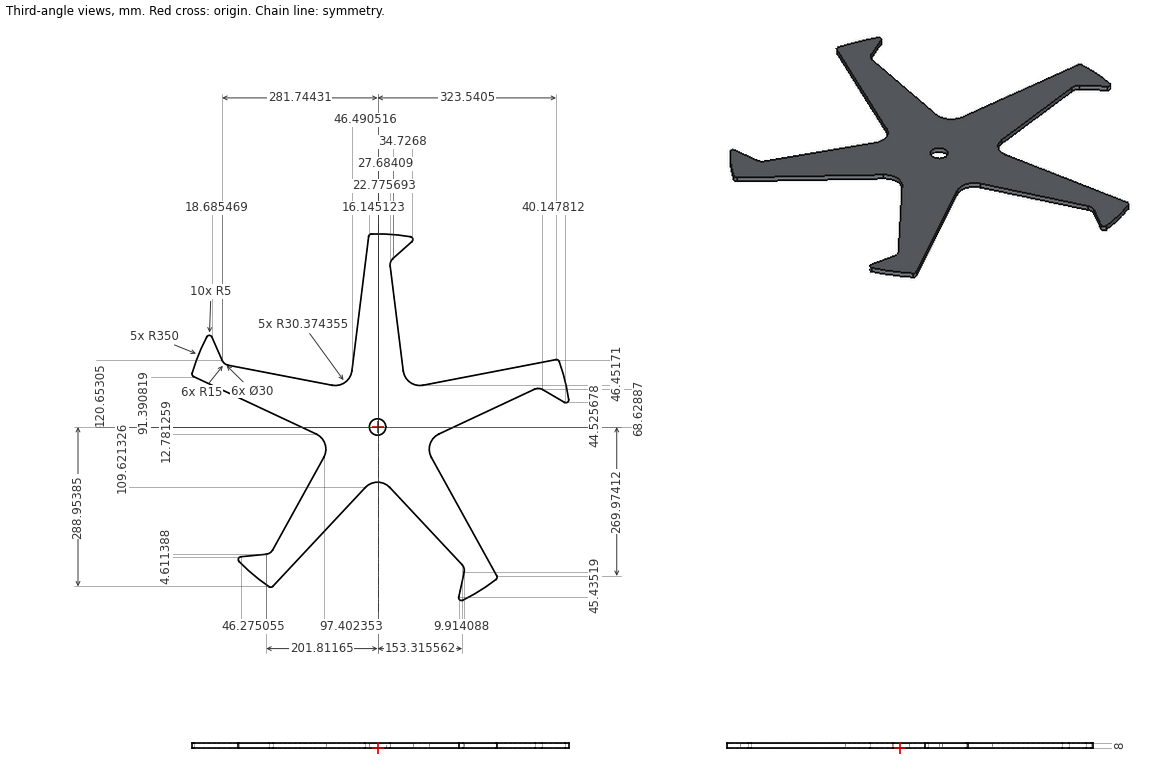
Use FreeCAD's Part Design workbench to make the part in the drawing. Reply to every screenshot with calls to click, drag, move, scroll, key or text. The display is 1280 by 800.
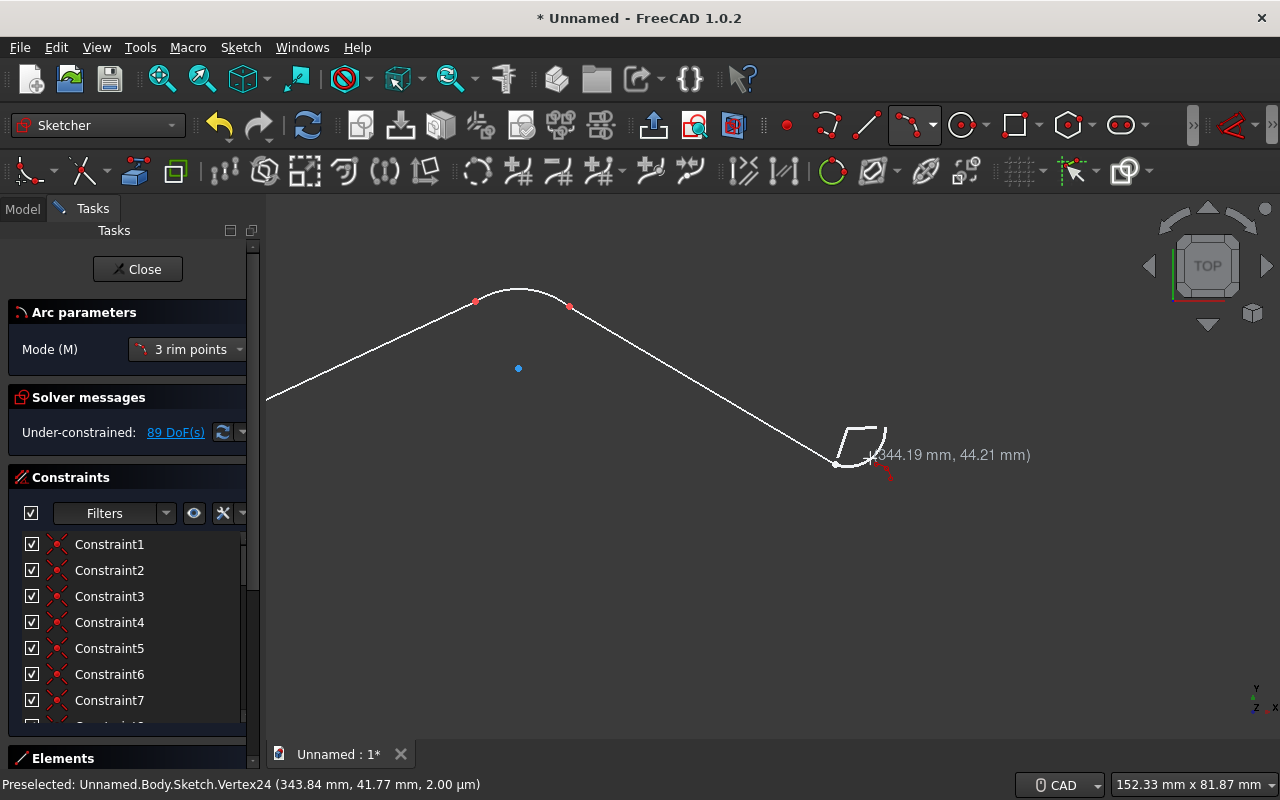
click(869, 457)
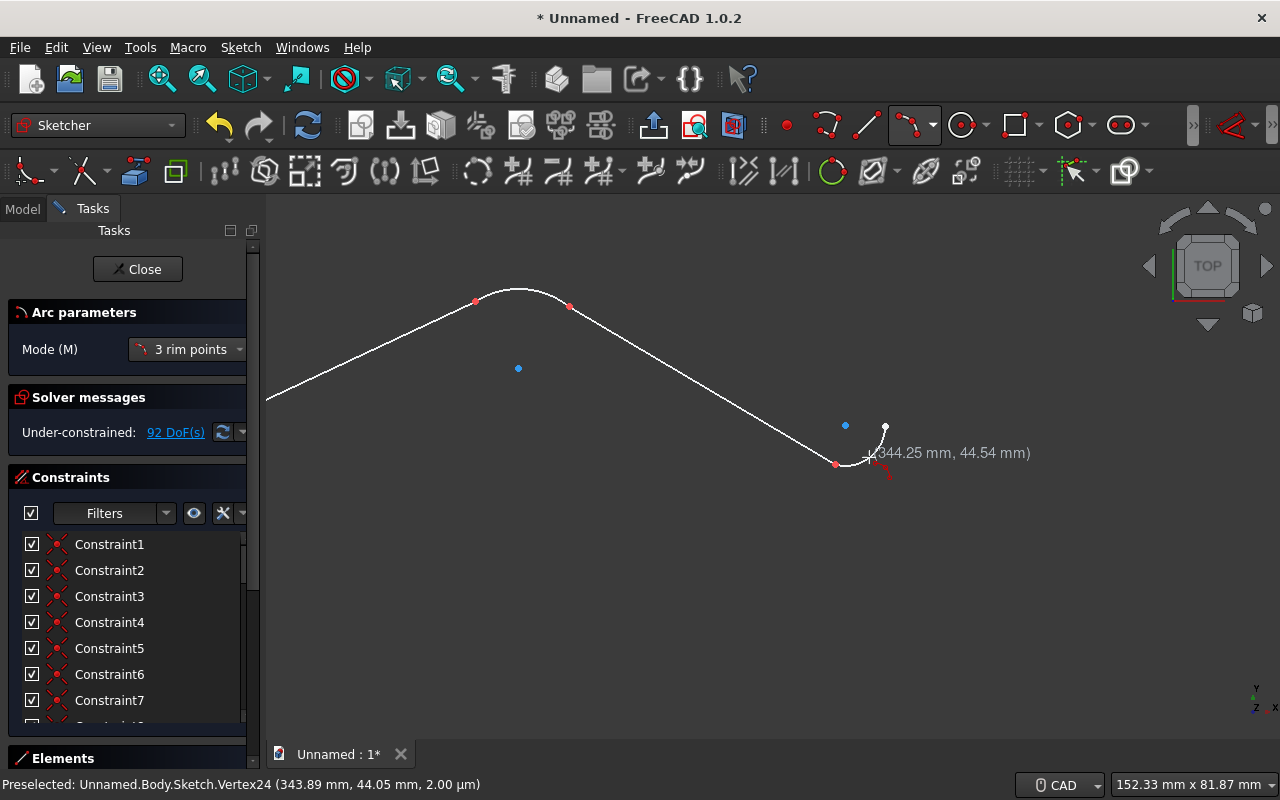
click(885, 427)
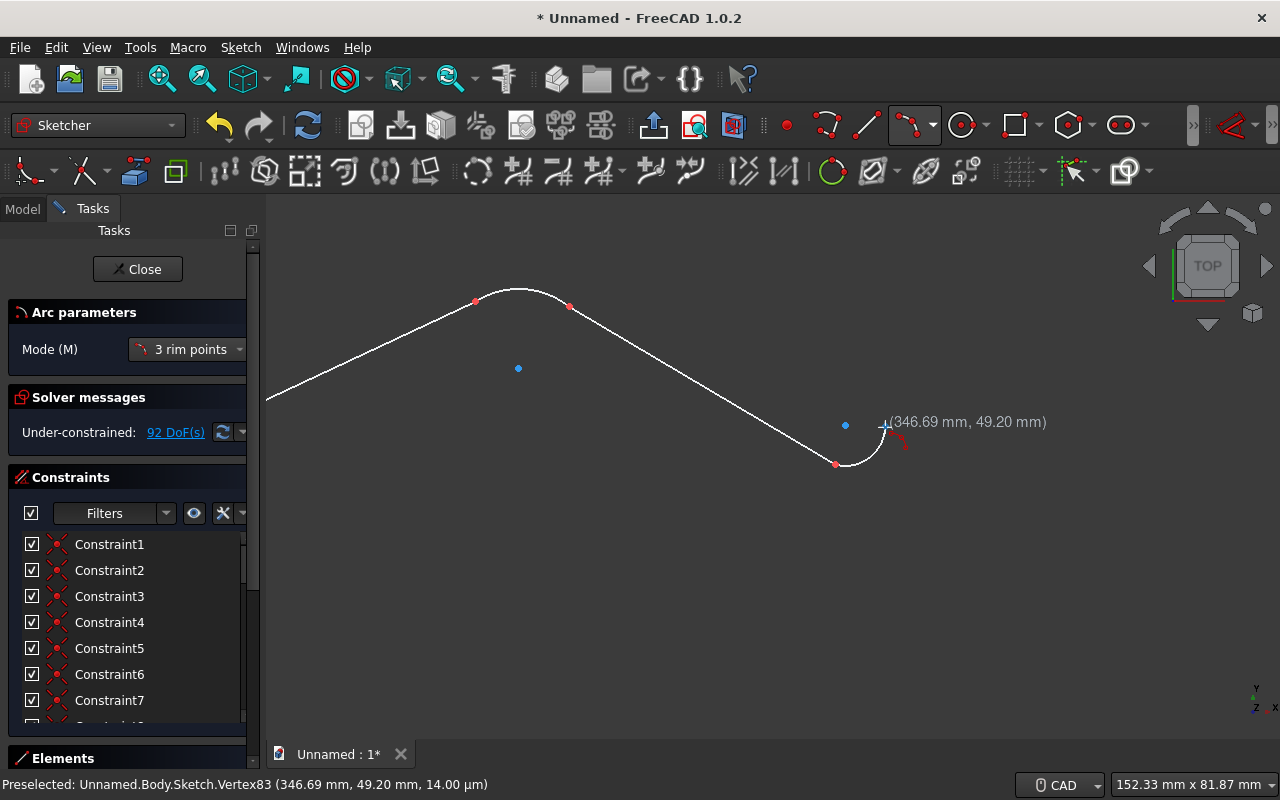
scroll(872, 453, down, 13)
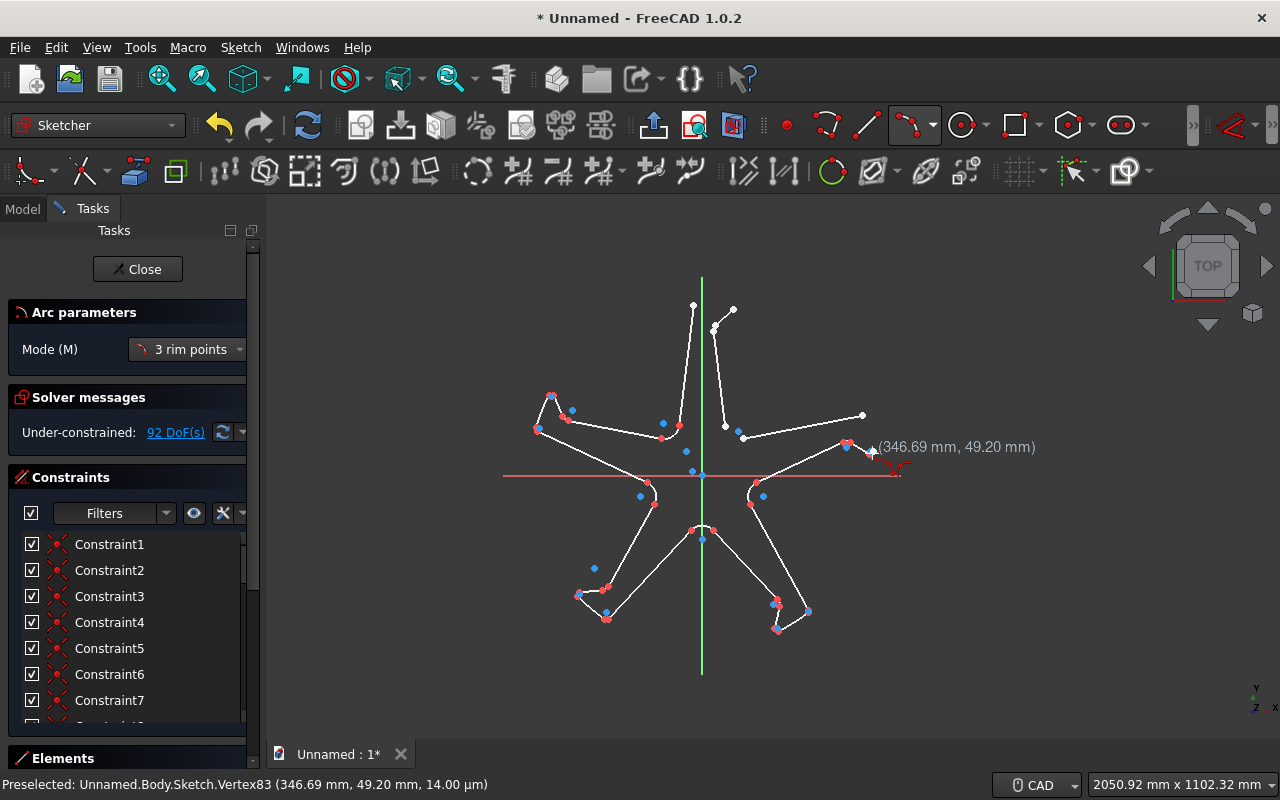
scroll(865, 417, up, 8)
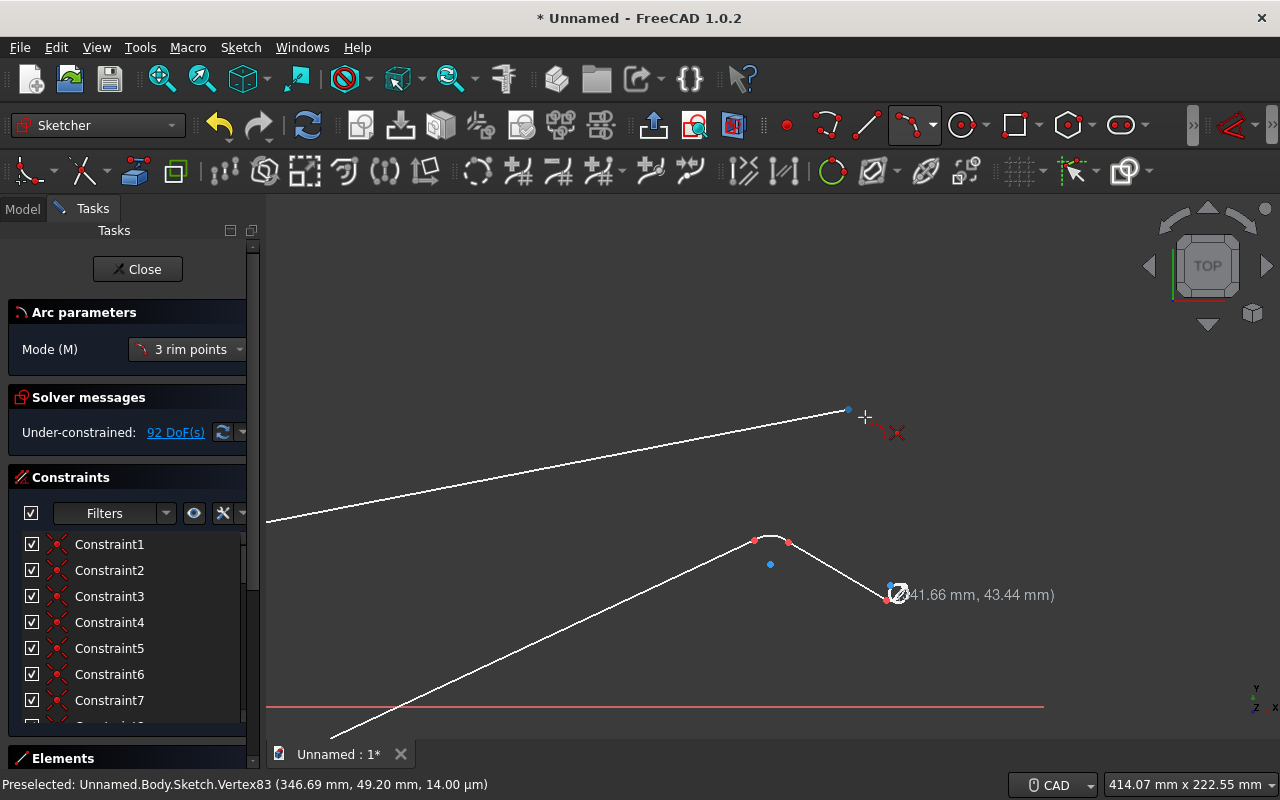
click(862, 416)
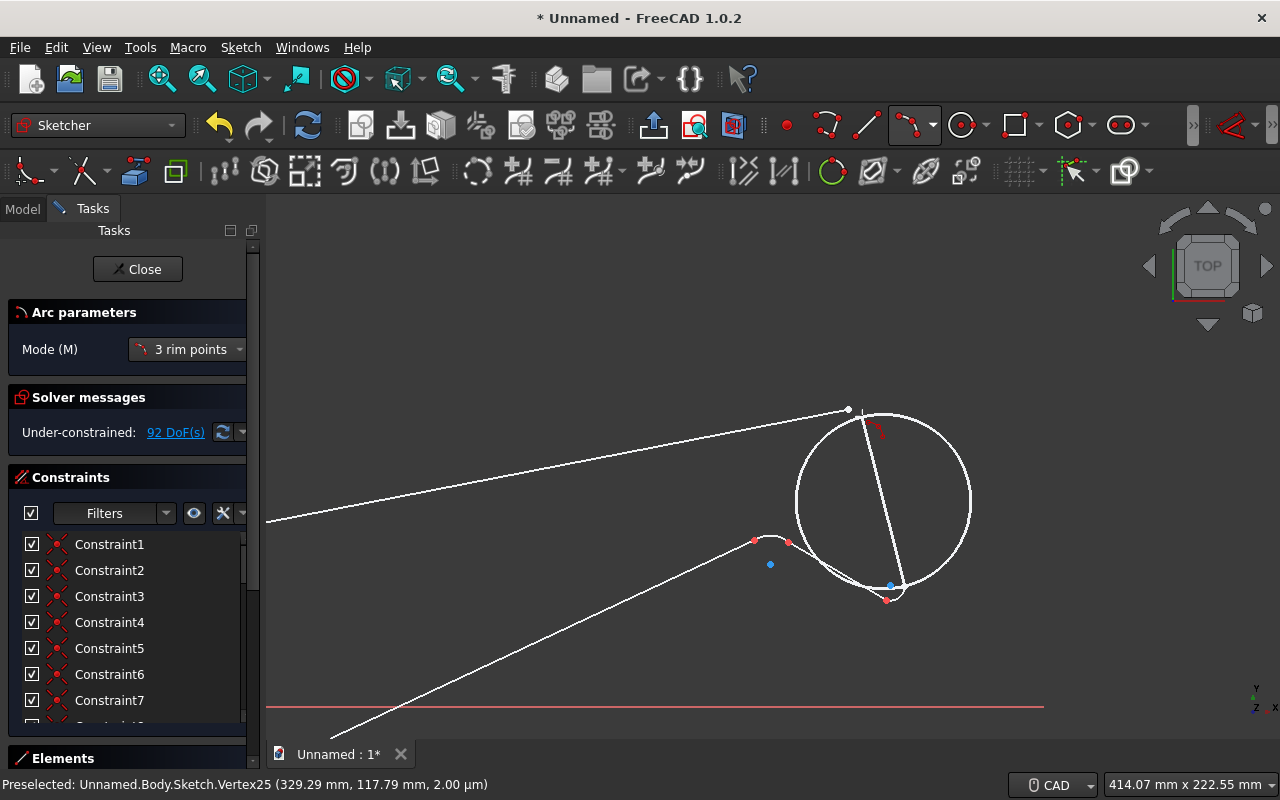
scroll(888, 499, up, 7)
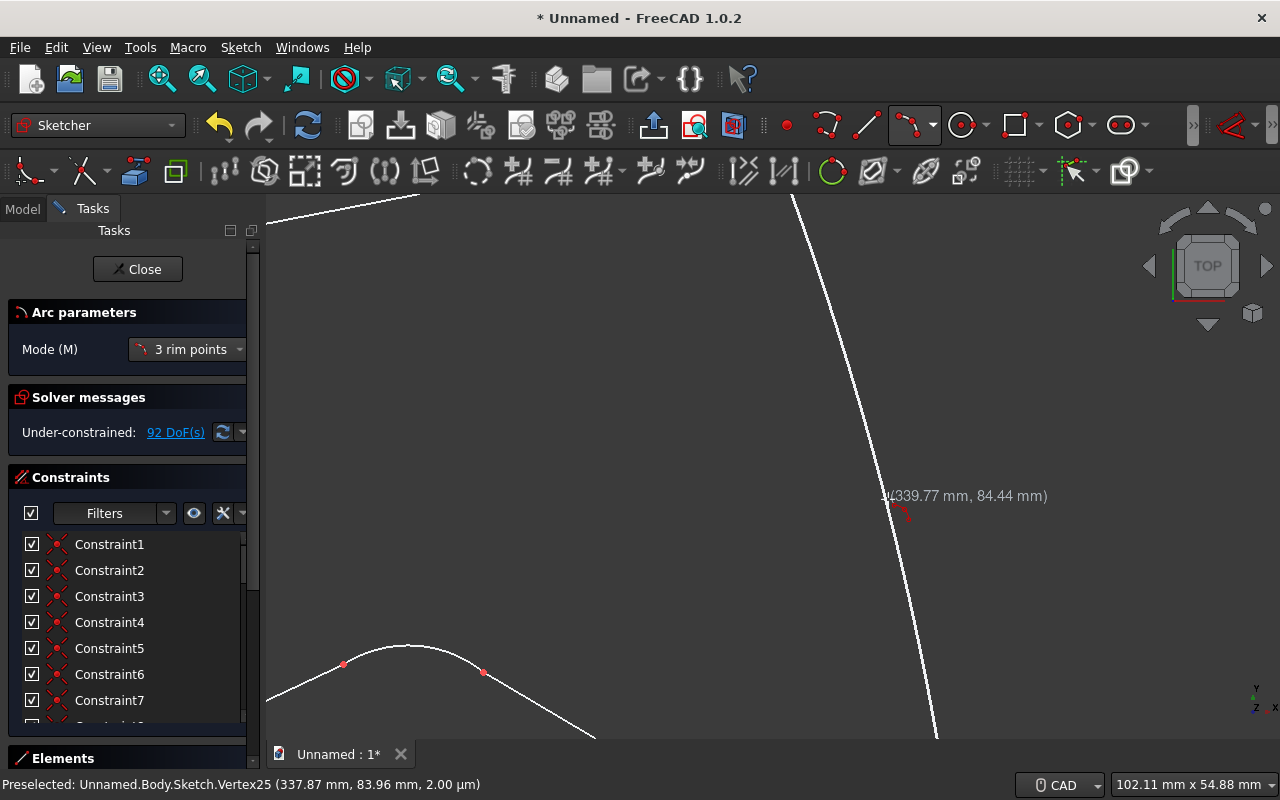
click(884, 499)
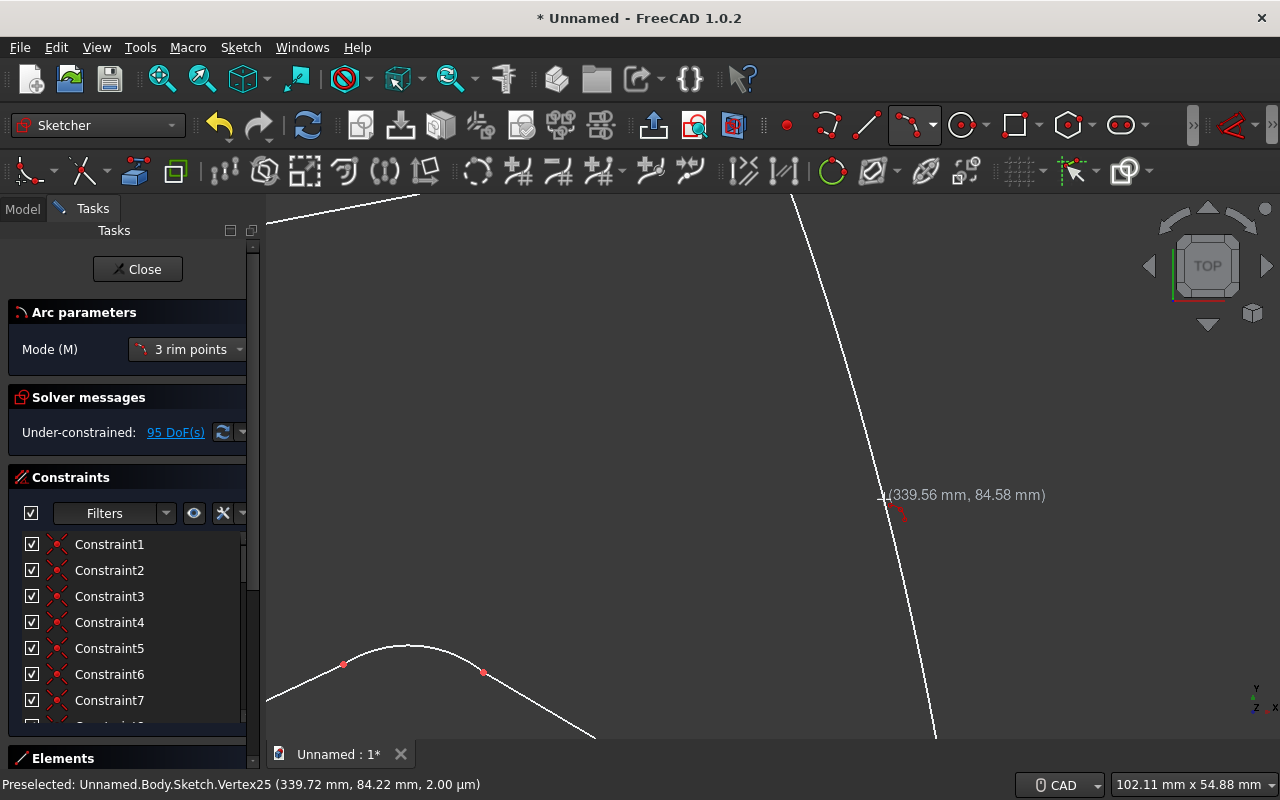
scroll(869, 430, down, 15)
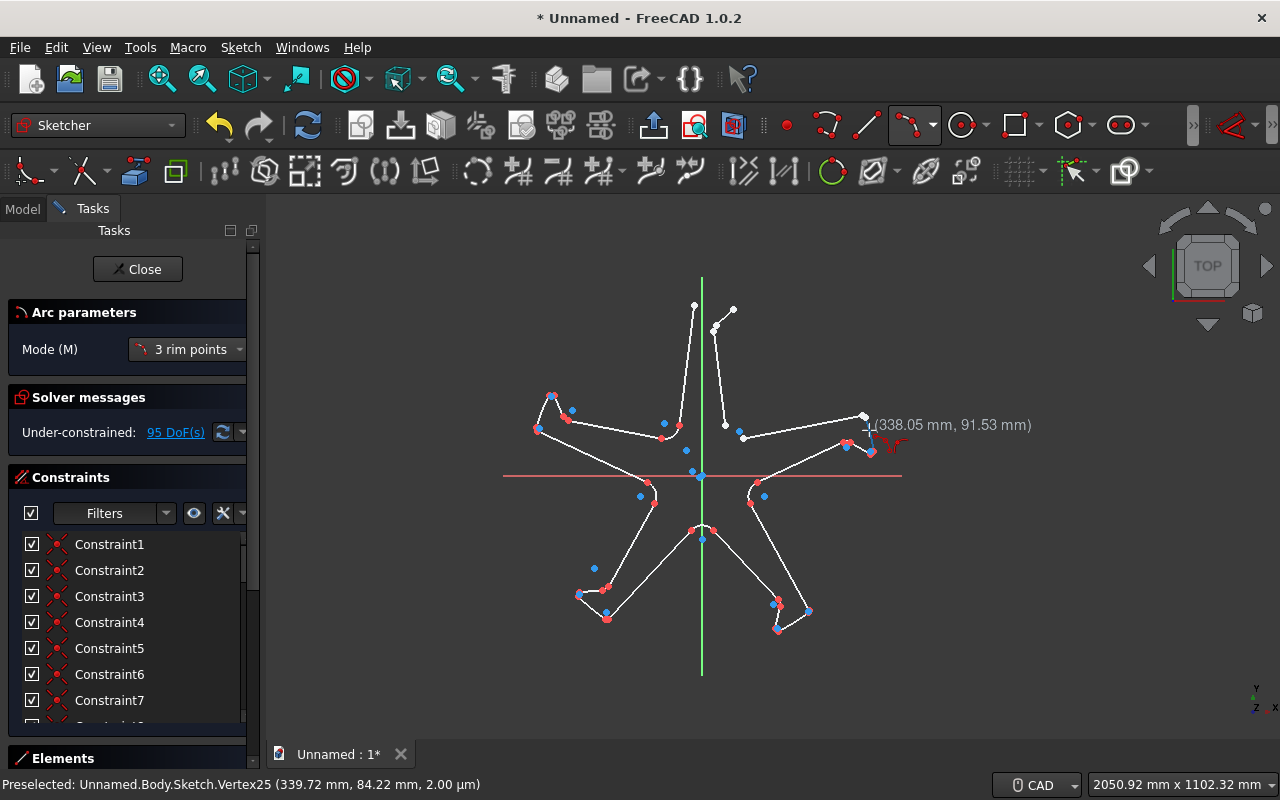
scroll(865, 417, up, 8)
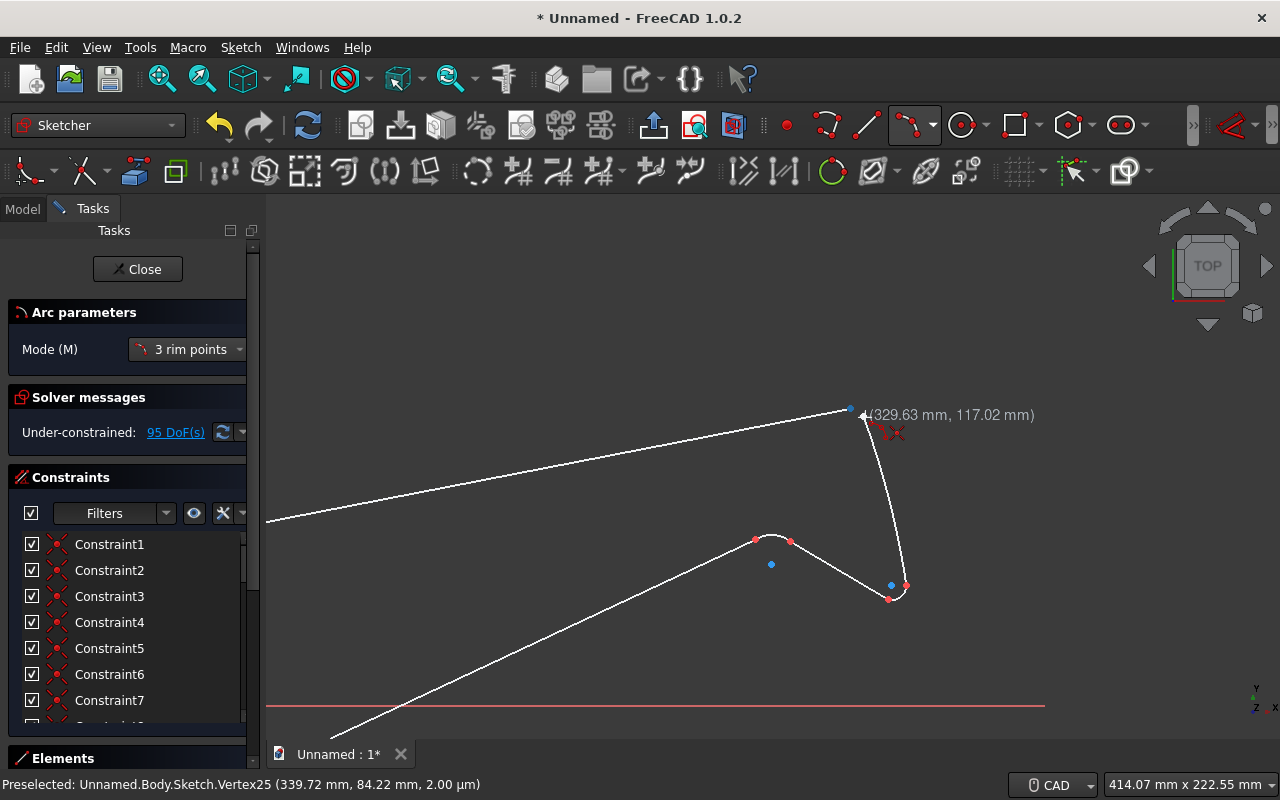
click(863, 416)
click(850, 409)